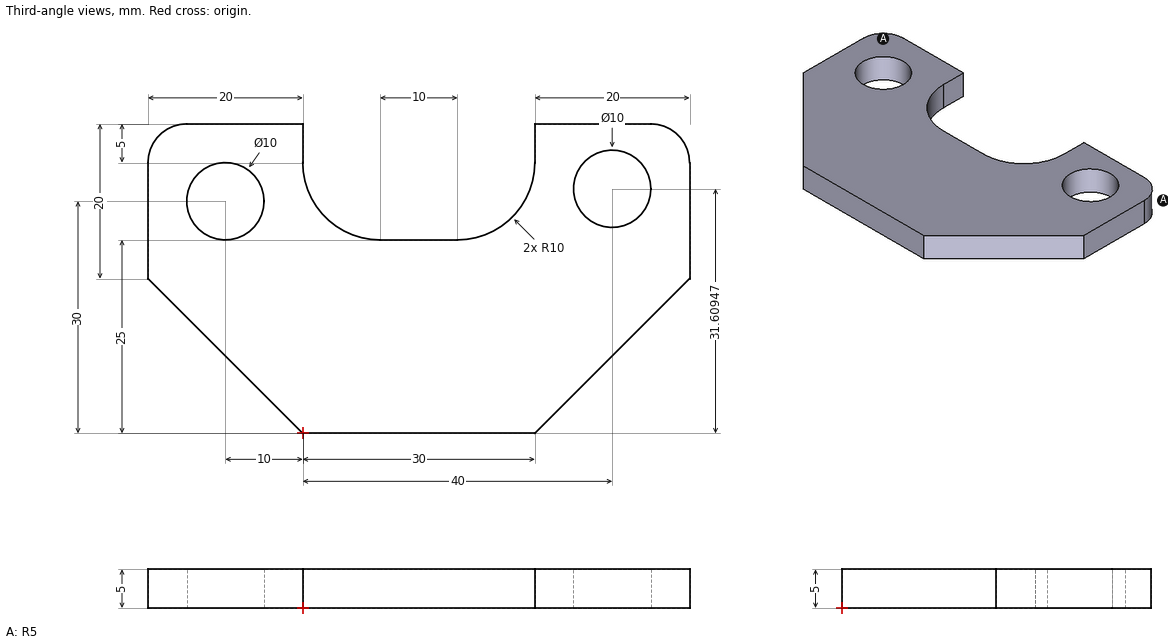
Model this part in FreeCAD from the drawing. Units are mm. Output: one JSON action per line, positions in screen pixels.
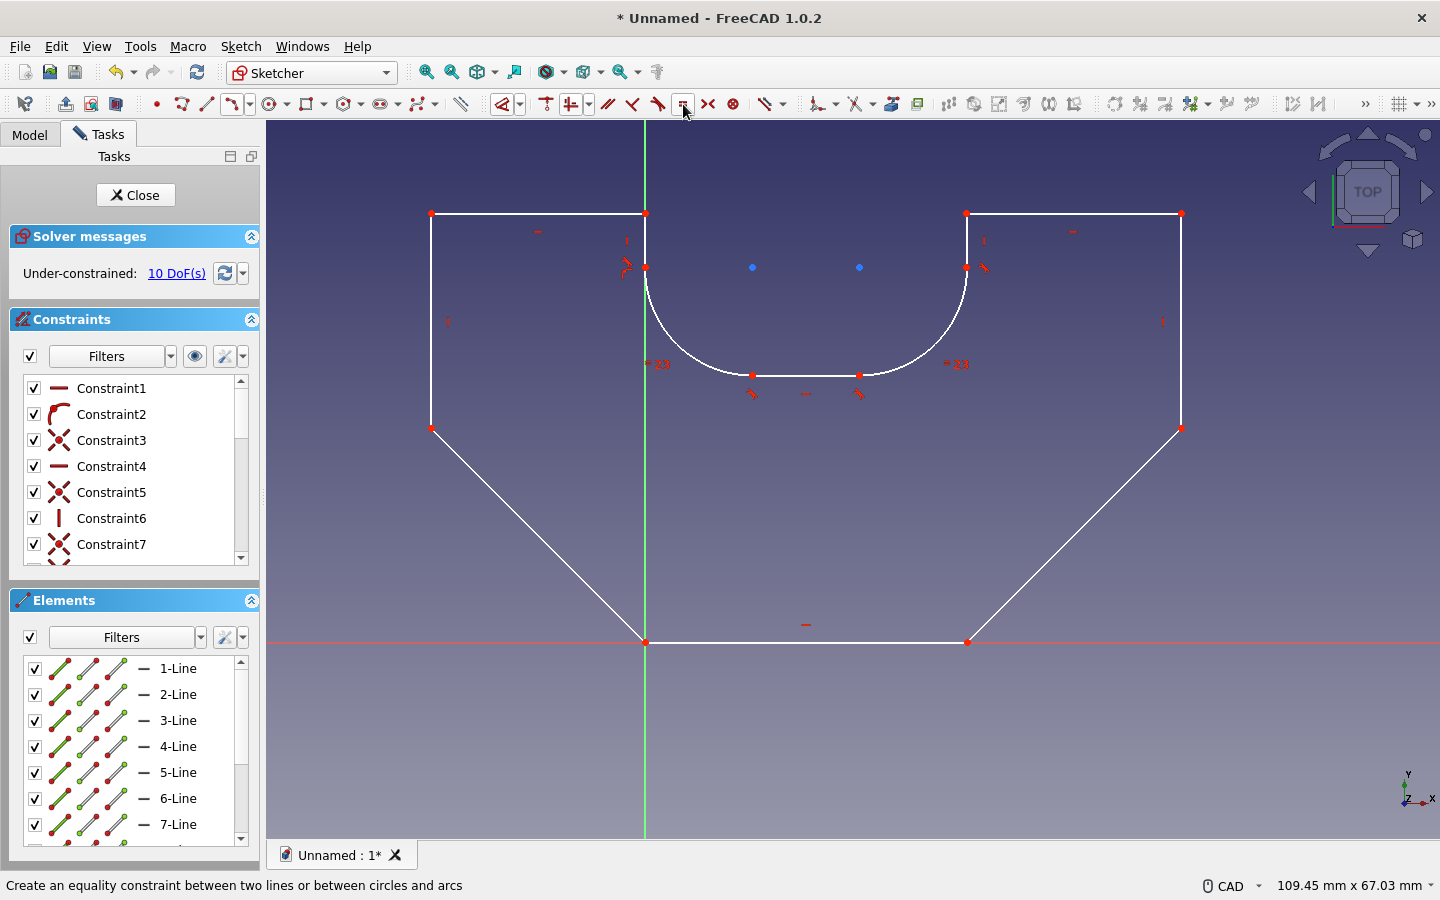
{"action": "left_click", "coordinate": [657, 317]}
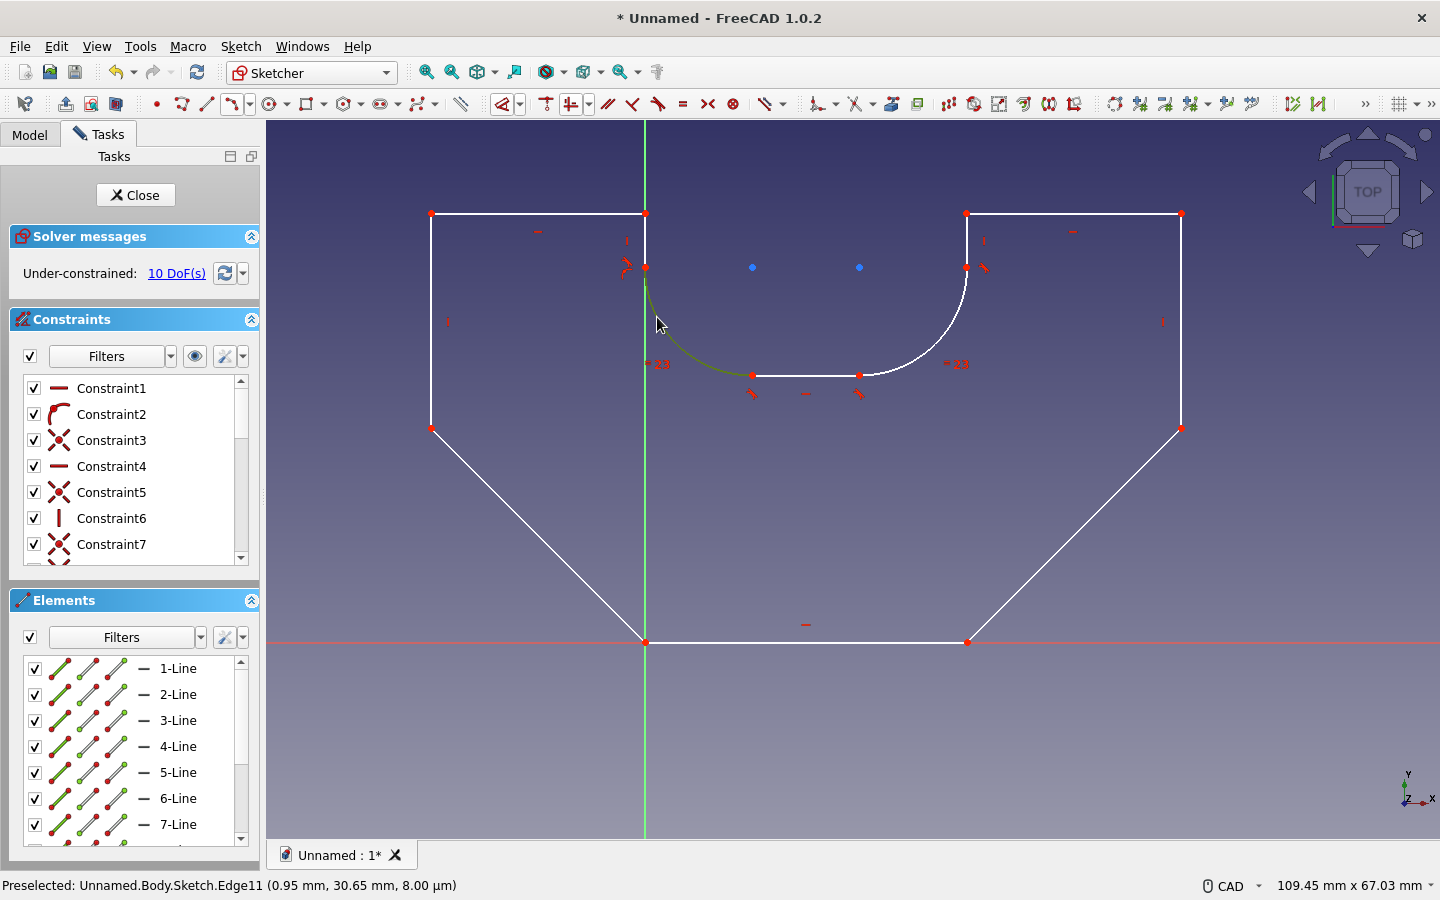
{"action": "key", "text": "k r"}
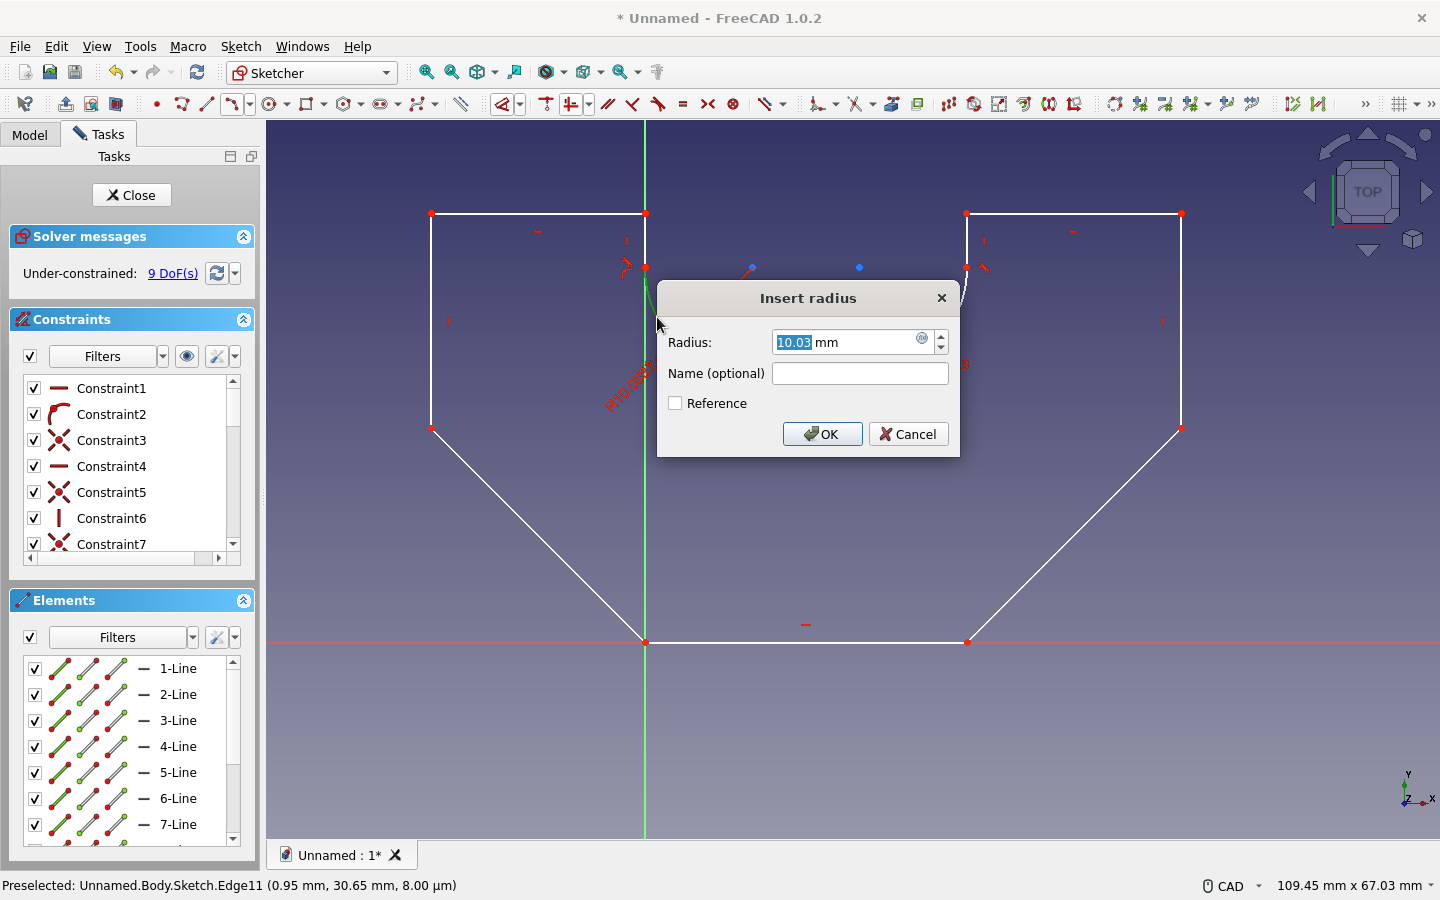
{"action": "type", "text": "10"}
{"action": "key", "text": "Return"}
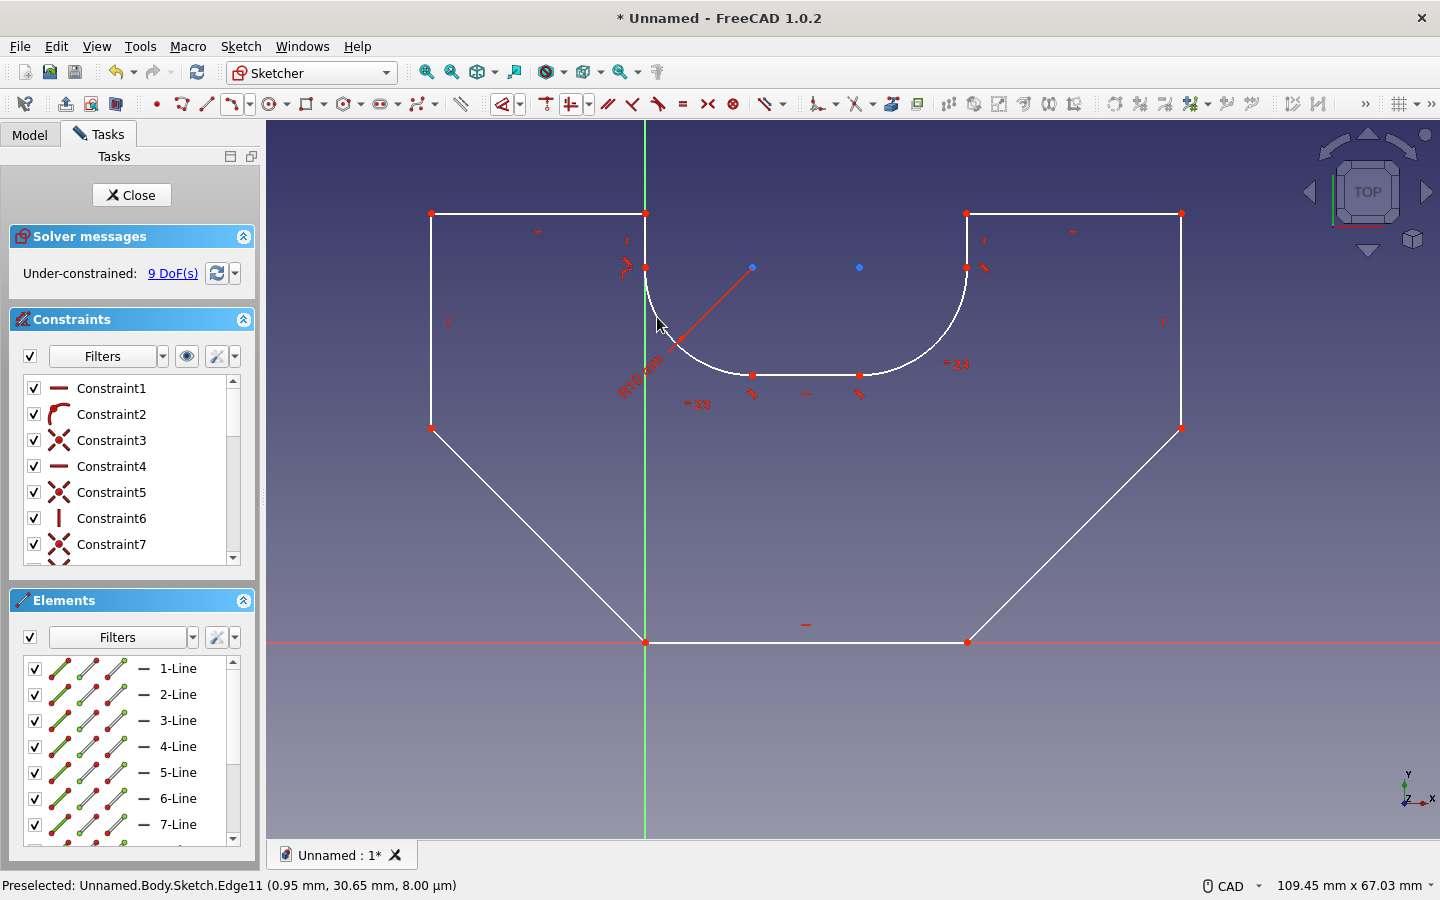
{"action": "left_click", "coordinate": [645, 252]}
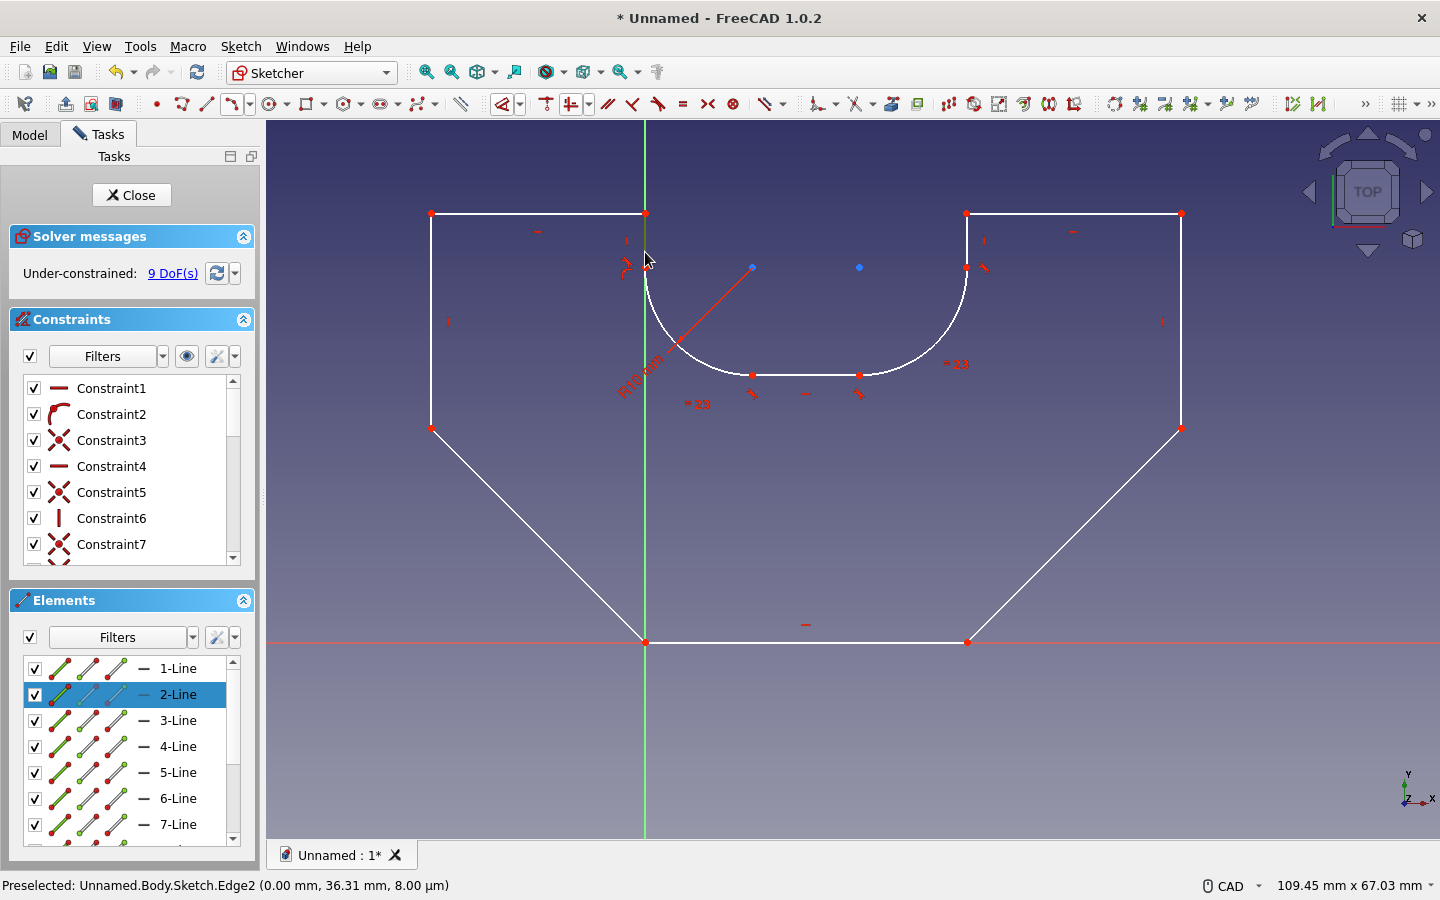
{"action": "left_click", "coordinate": [520, 104]}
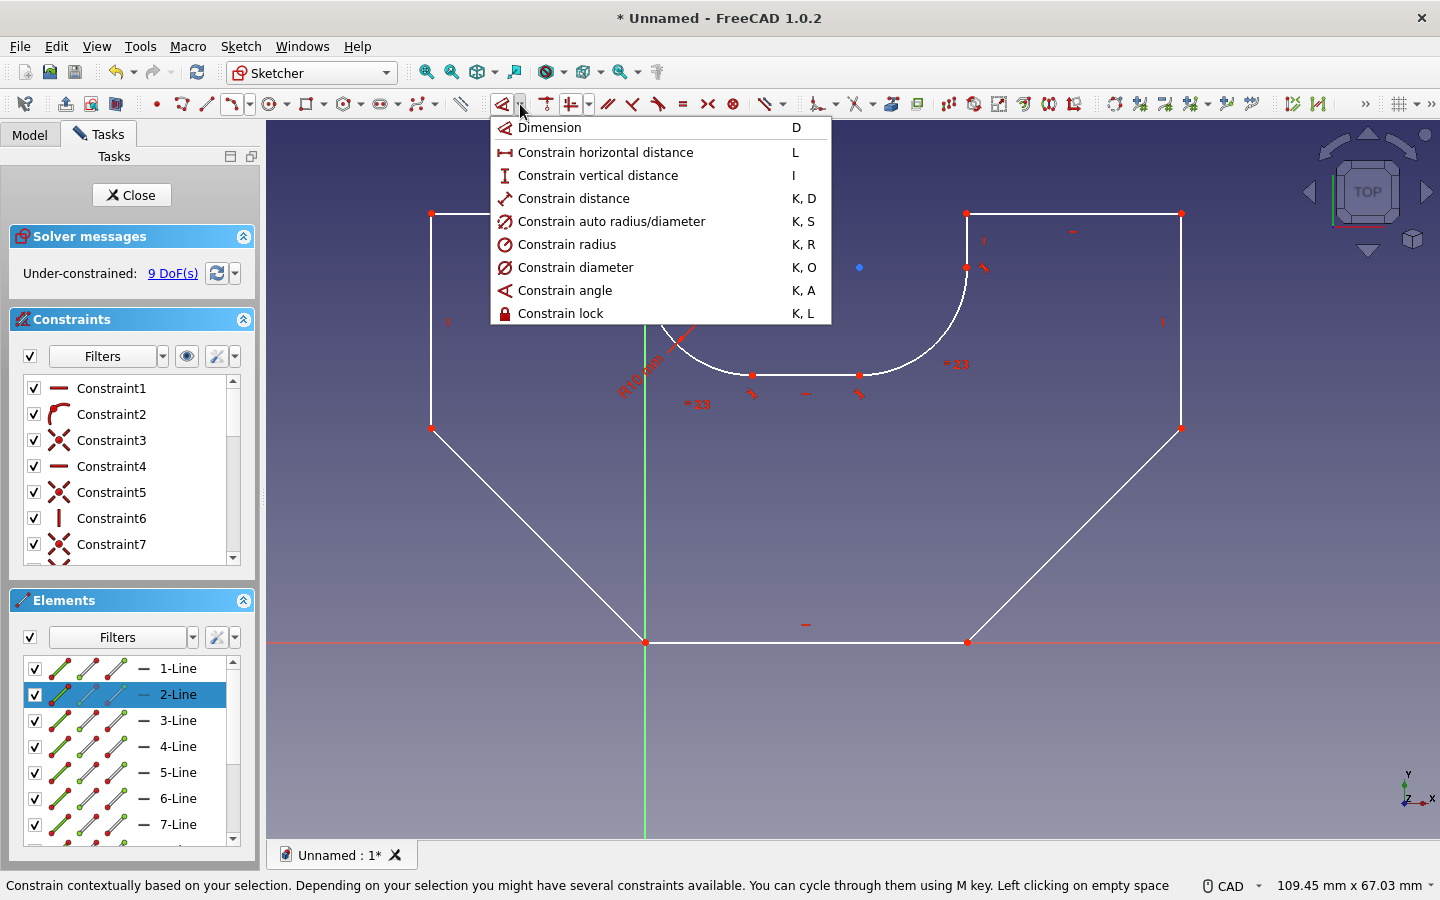
{"action": "left_click", "coordinate": [661, 176]}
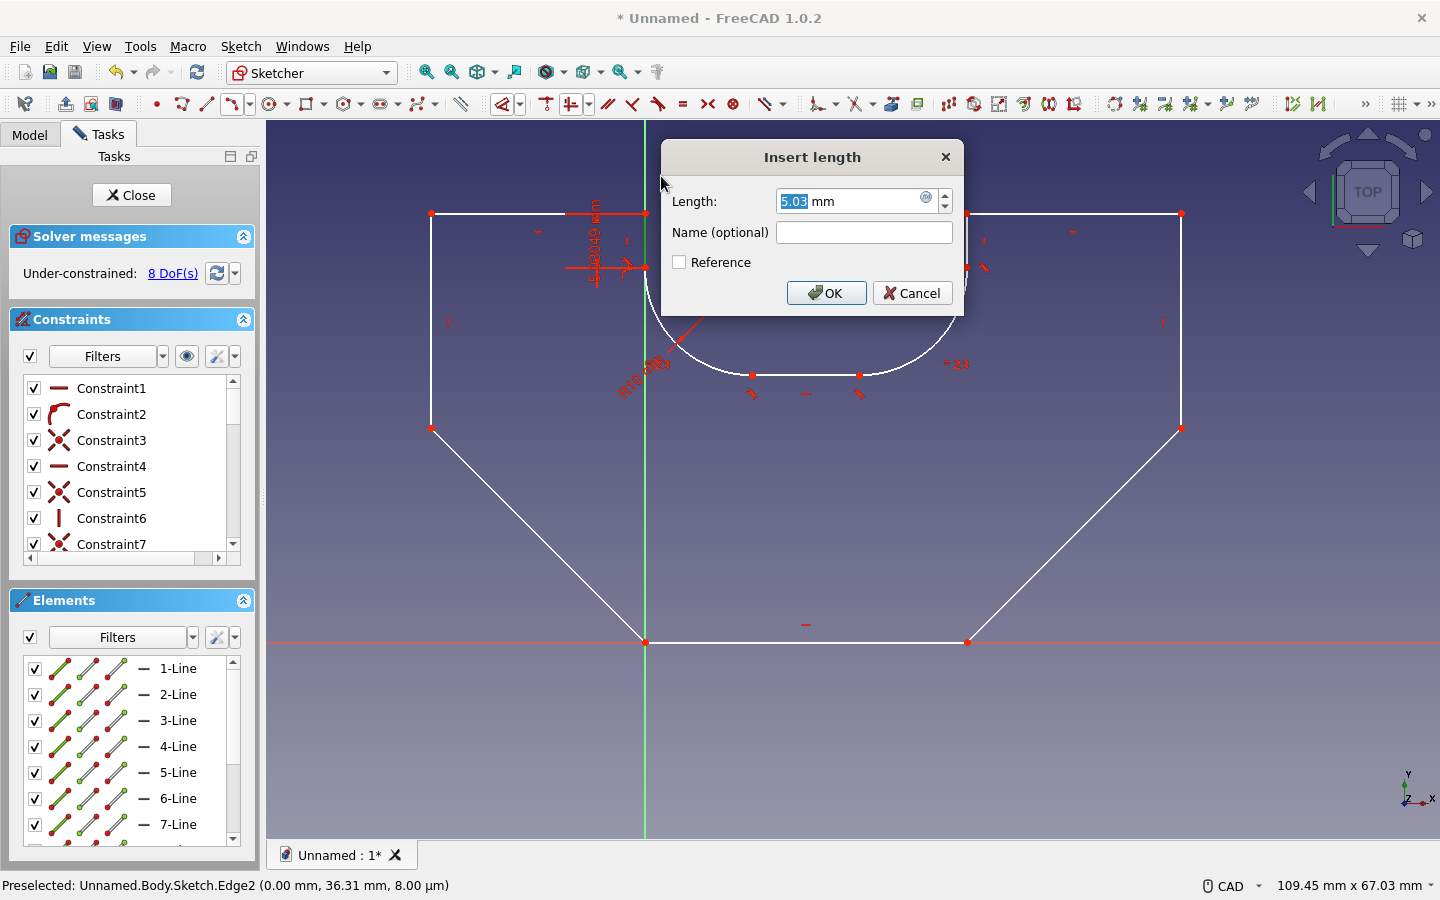
{"action": "type", "text": "5"}
{"action": "key", "text": "Return"}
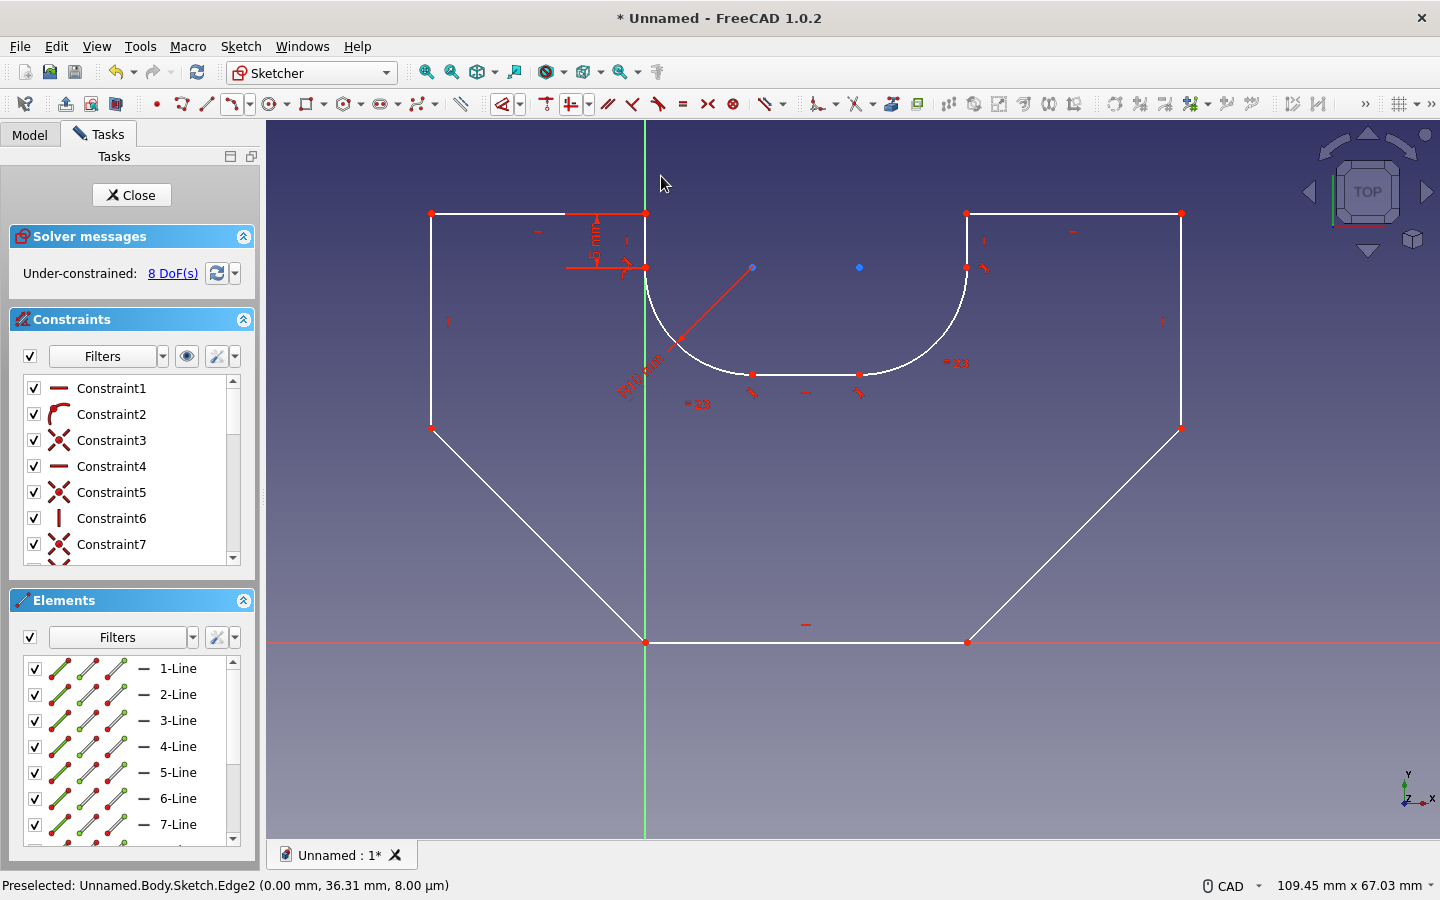
{"action": "left_click", "coordinate": [967, 230]}